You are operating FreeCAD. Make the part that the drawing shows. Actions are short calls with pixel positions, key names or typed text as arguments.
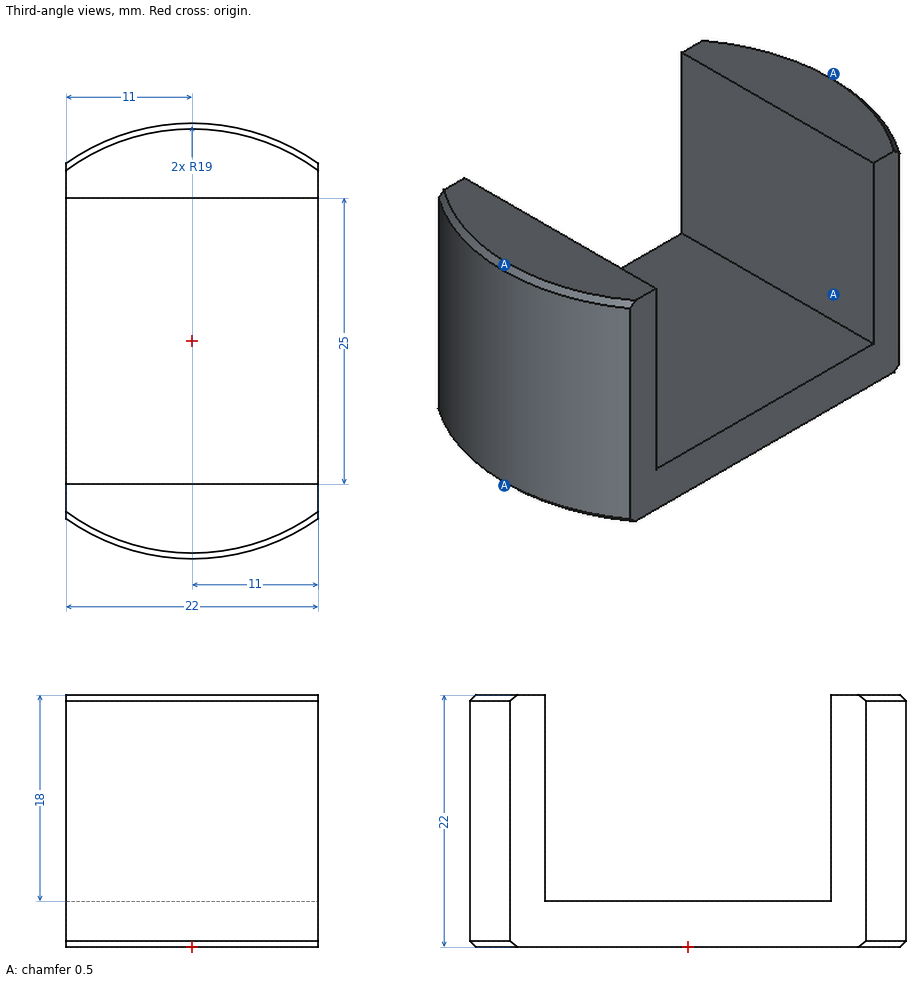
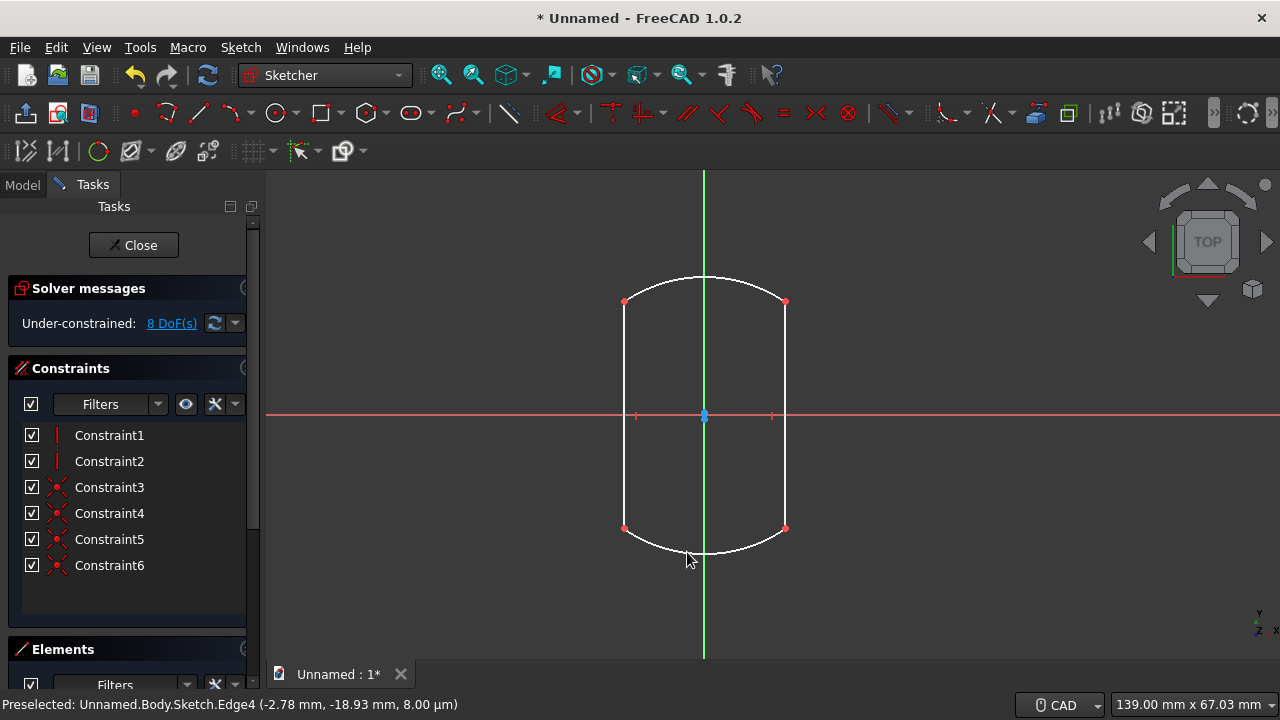
click(738, 281)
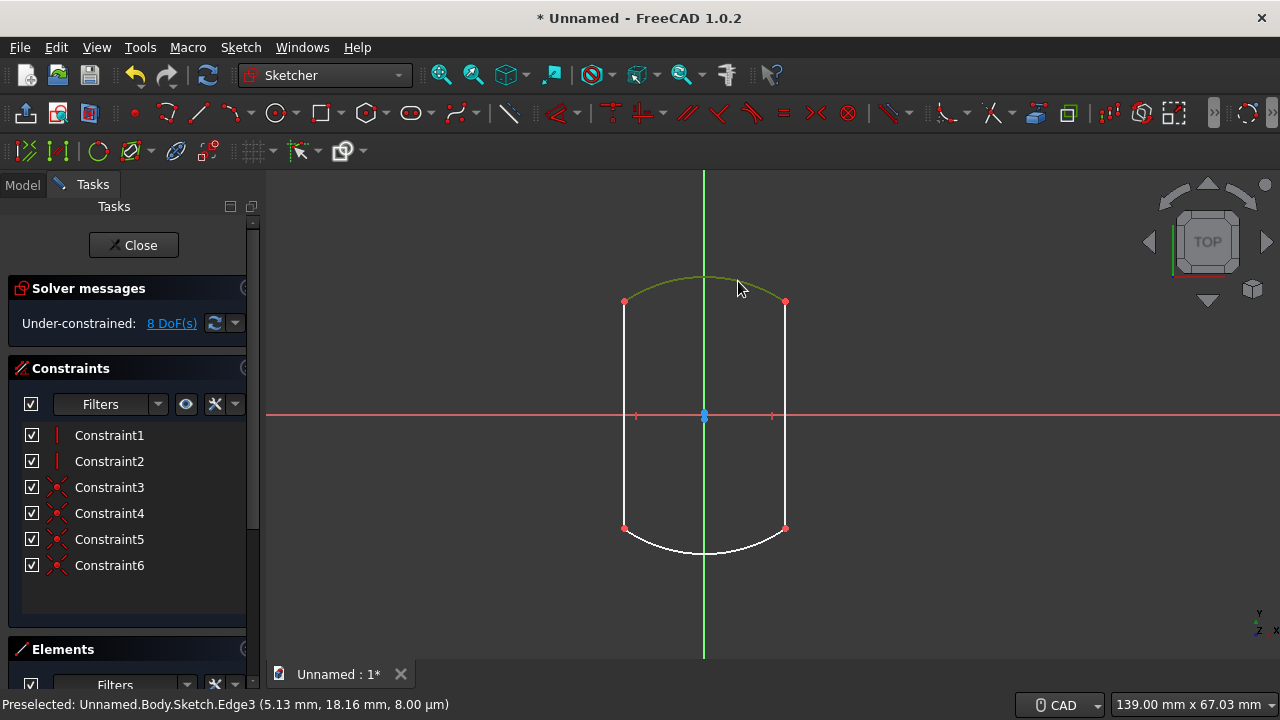
click(671, 550)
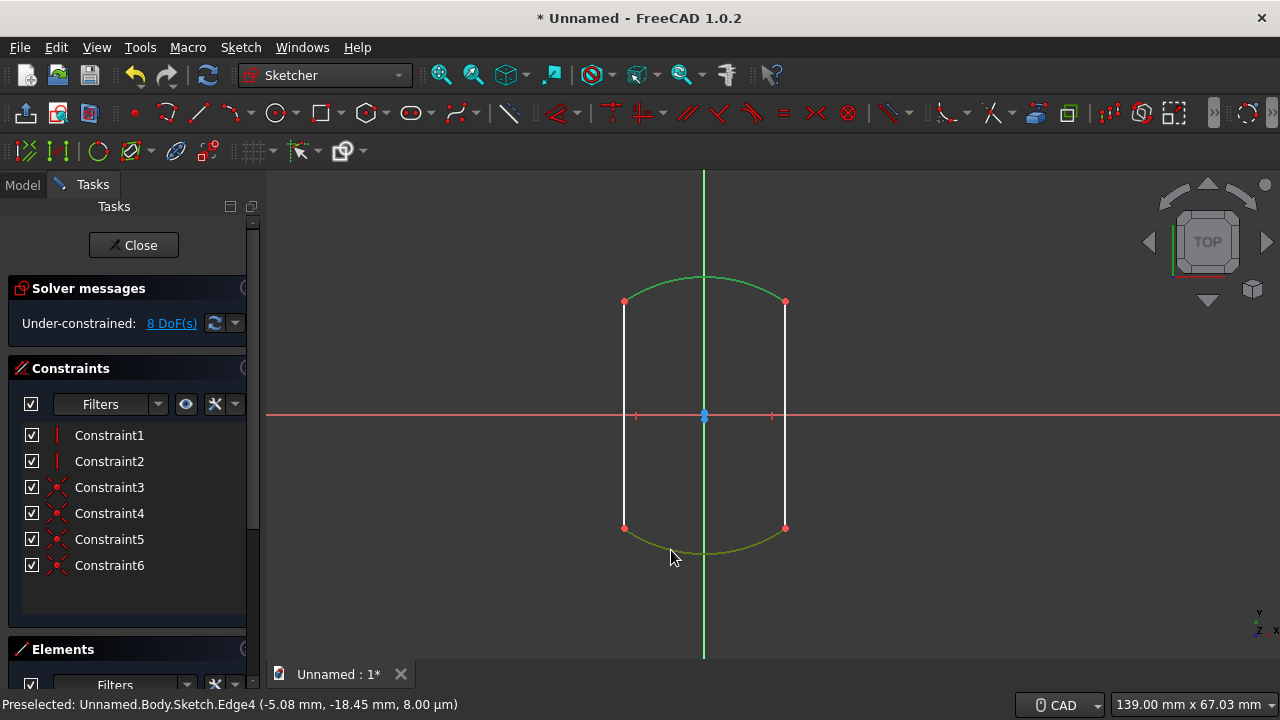
click(612, 114)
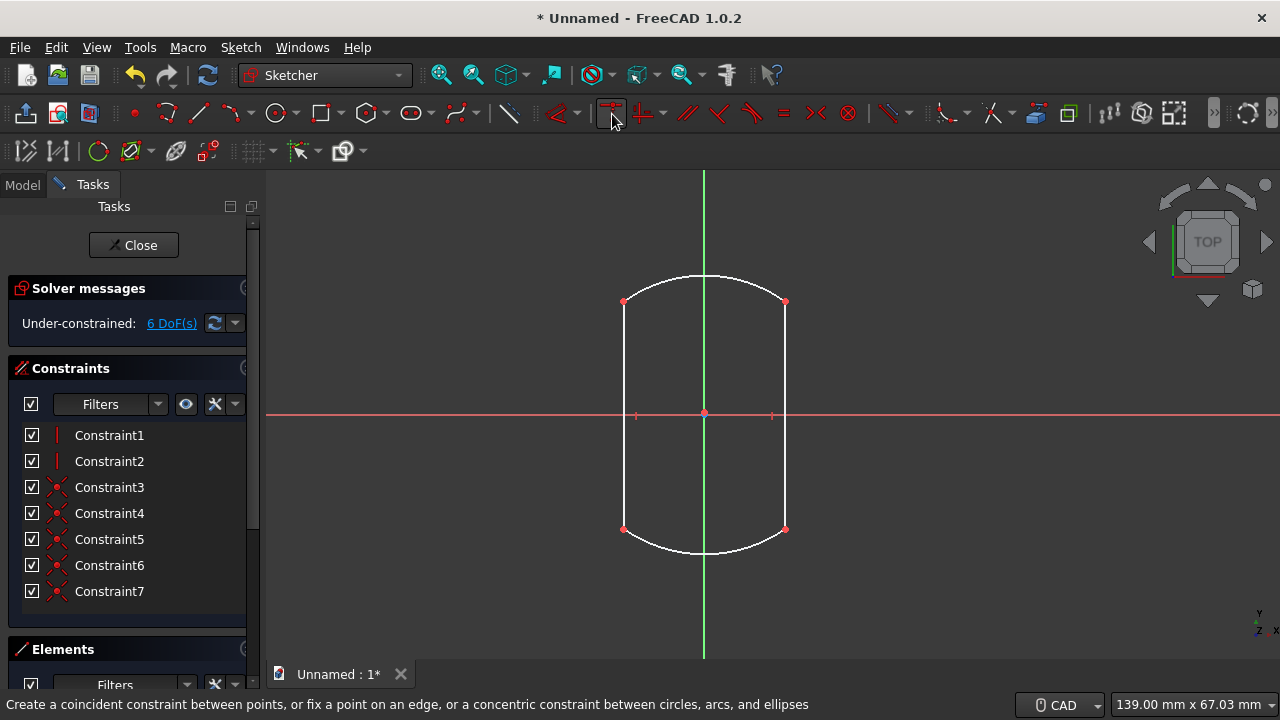
drag(694, 403, 715, 424)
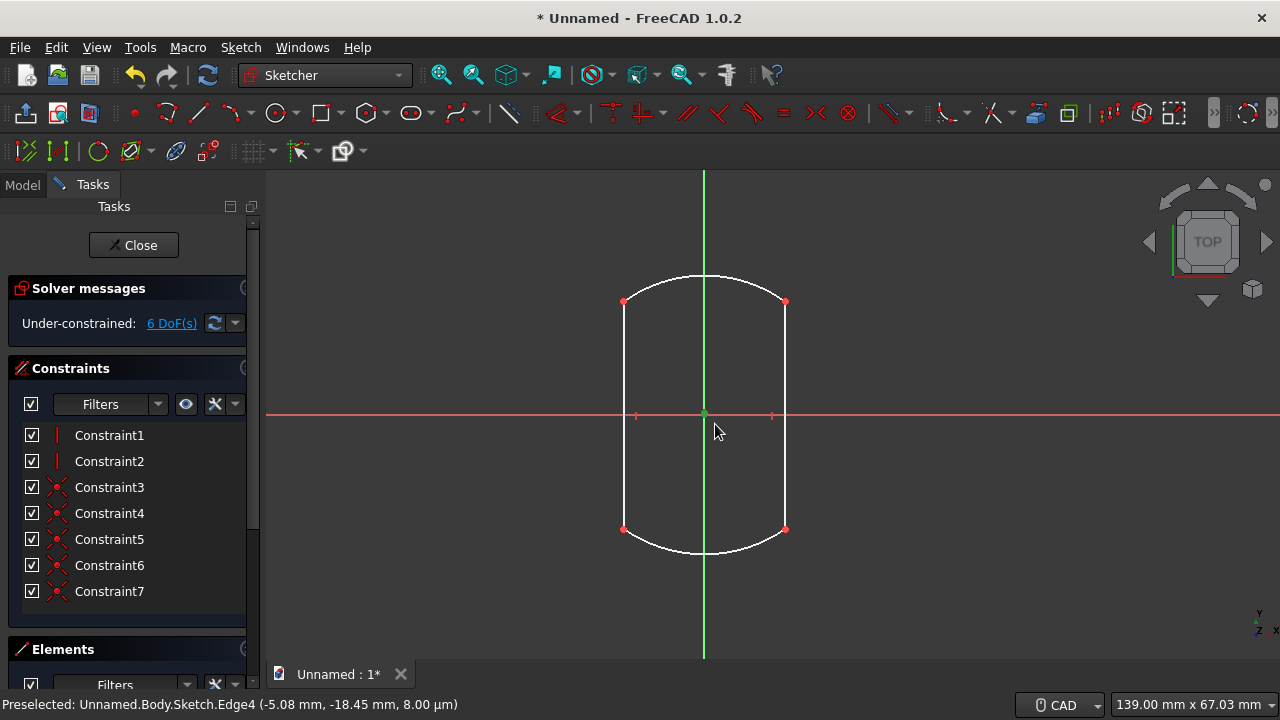
click(612, 114)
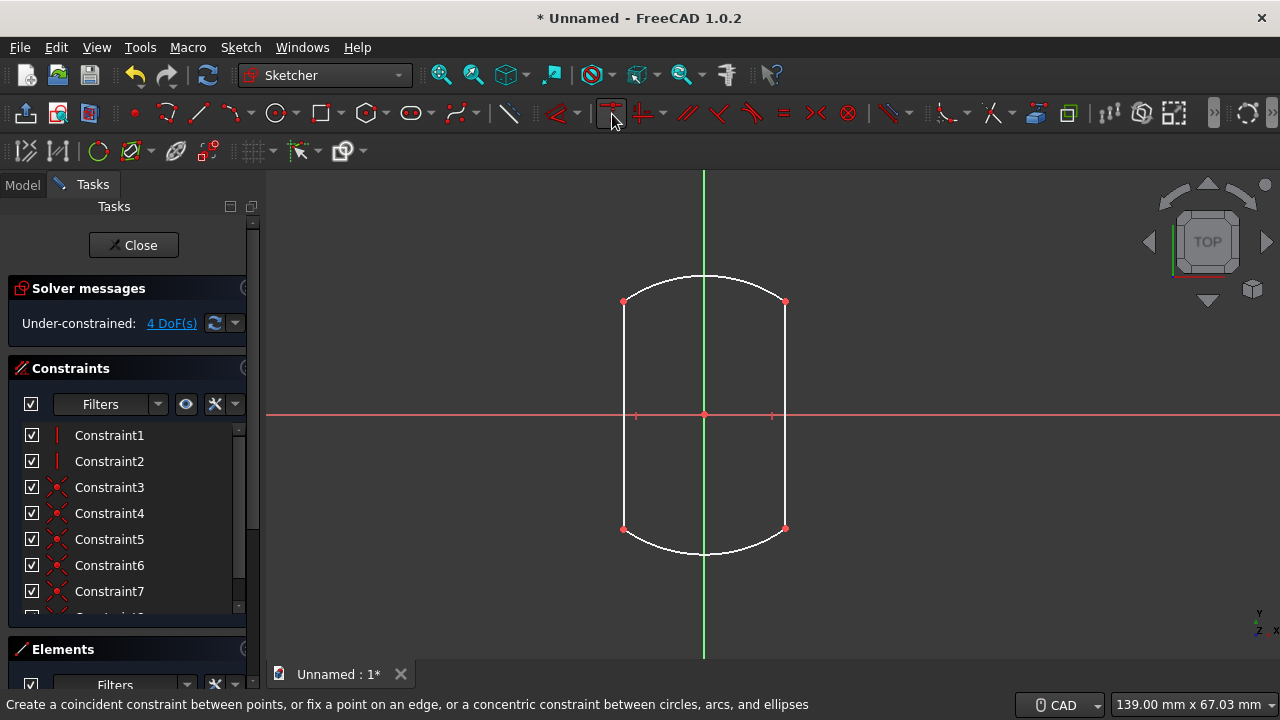
click(739, 280)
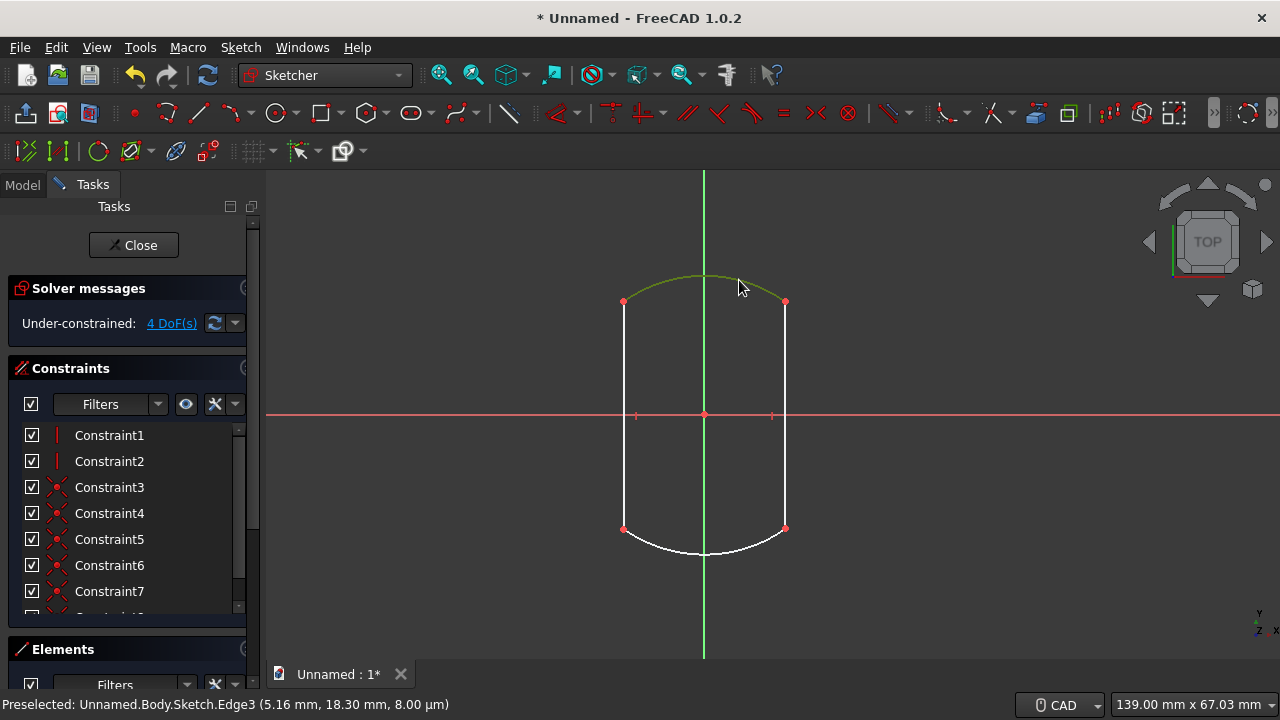
click(670, 550)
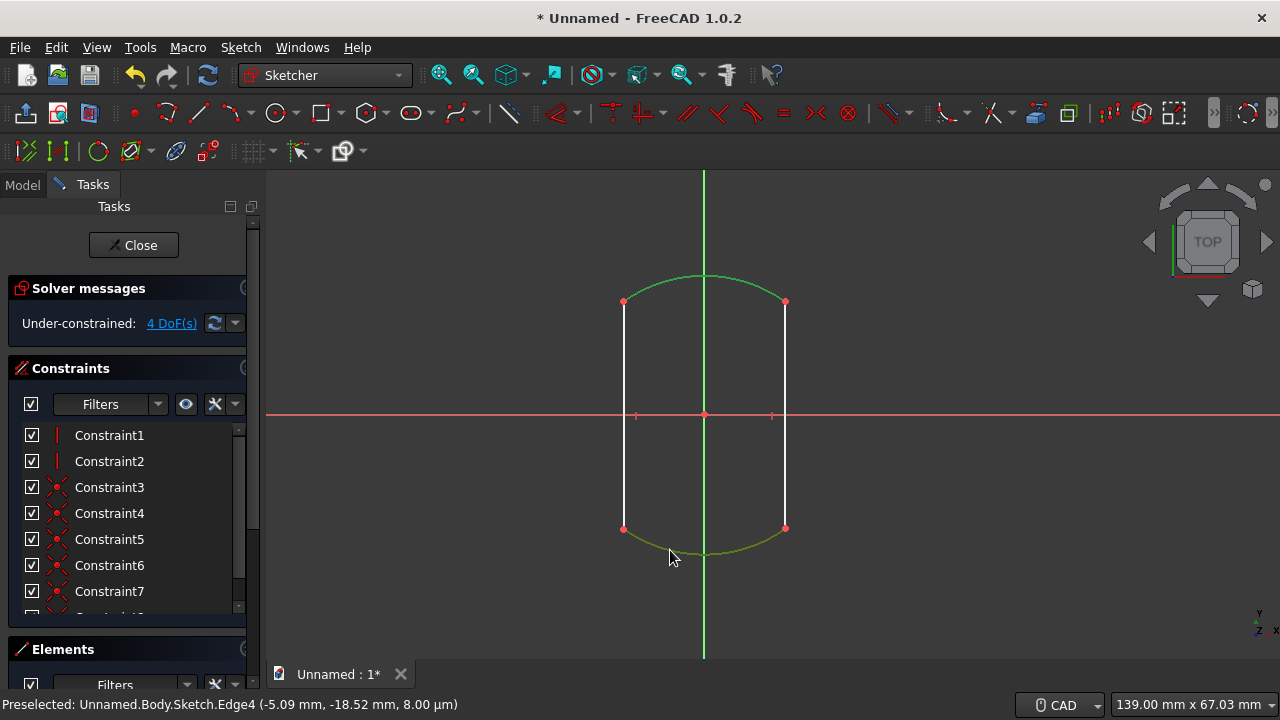
click(784, 114)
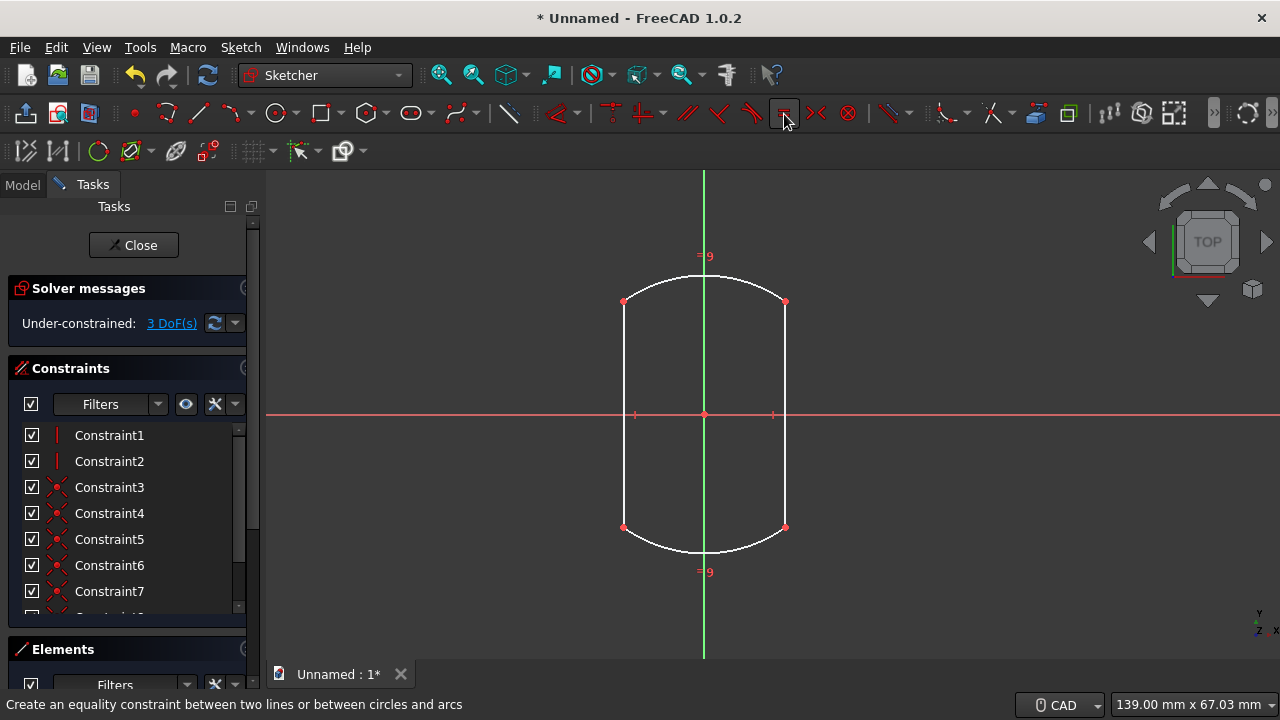
click(739, 280)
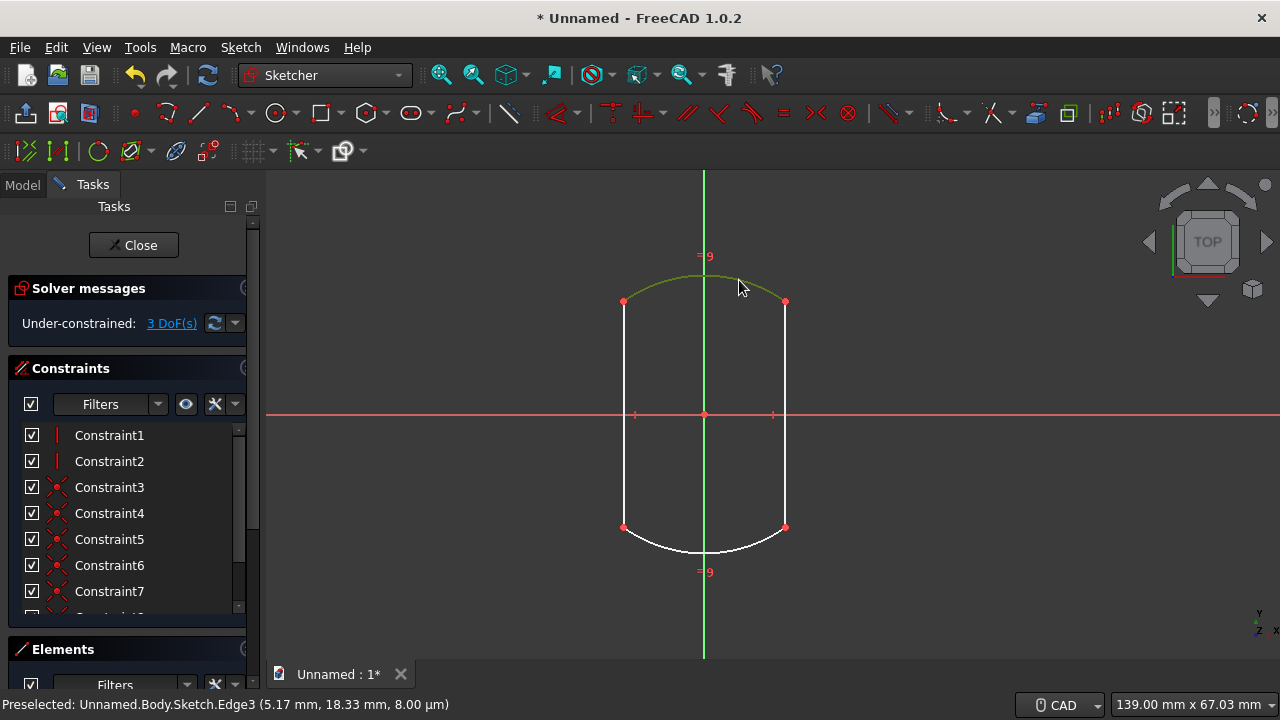
click(580, 114)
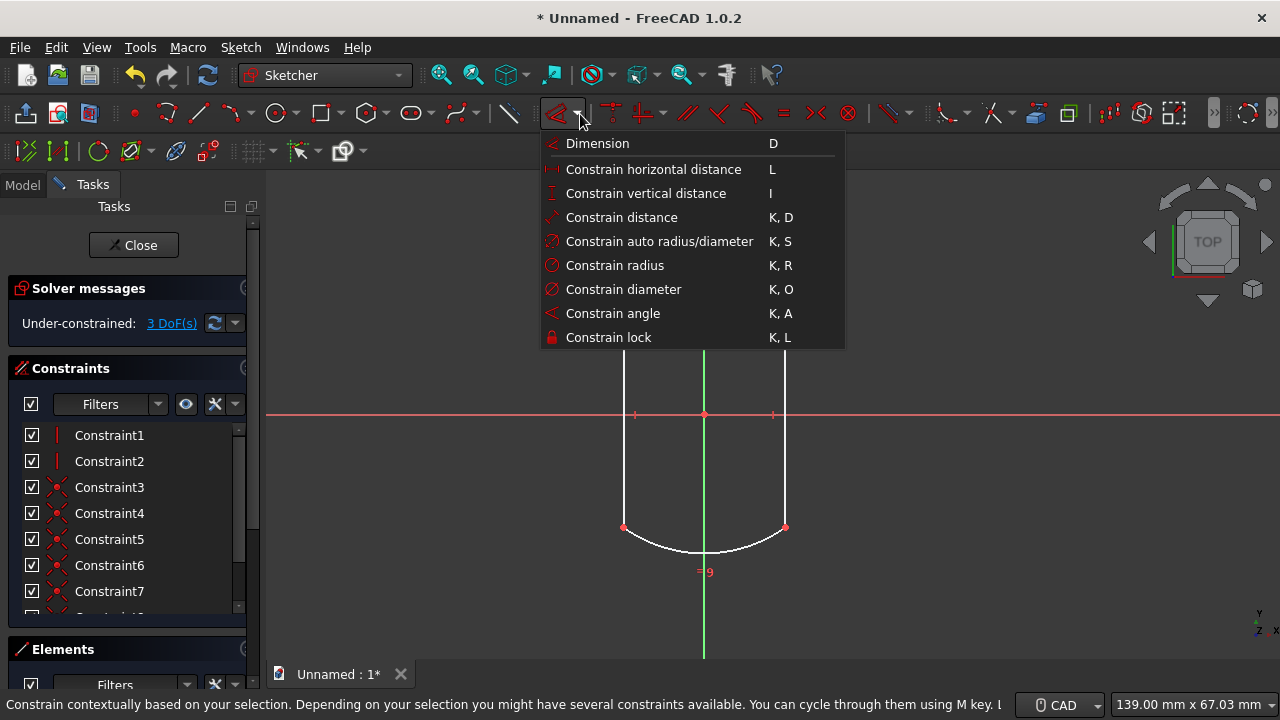
click(693, 265)